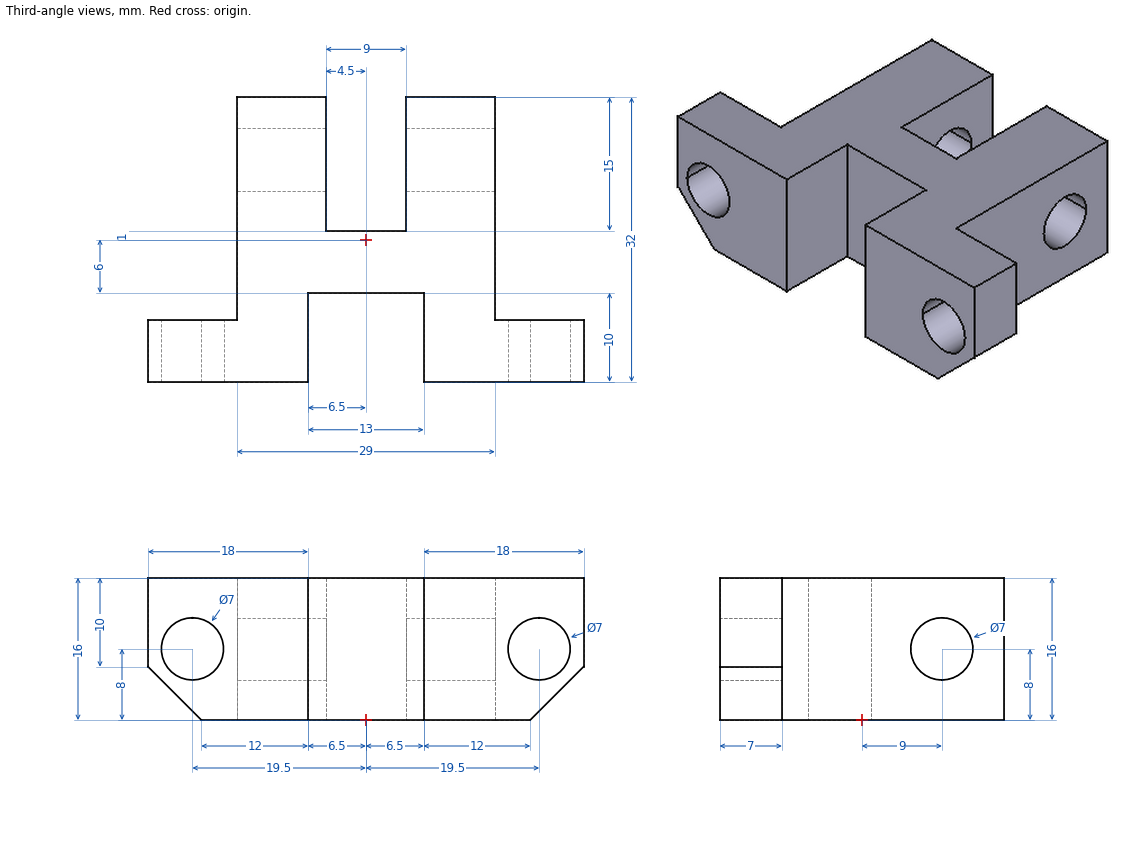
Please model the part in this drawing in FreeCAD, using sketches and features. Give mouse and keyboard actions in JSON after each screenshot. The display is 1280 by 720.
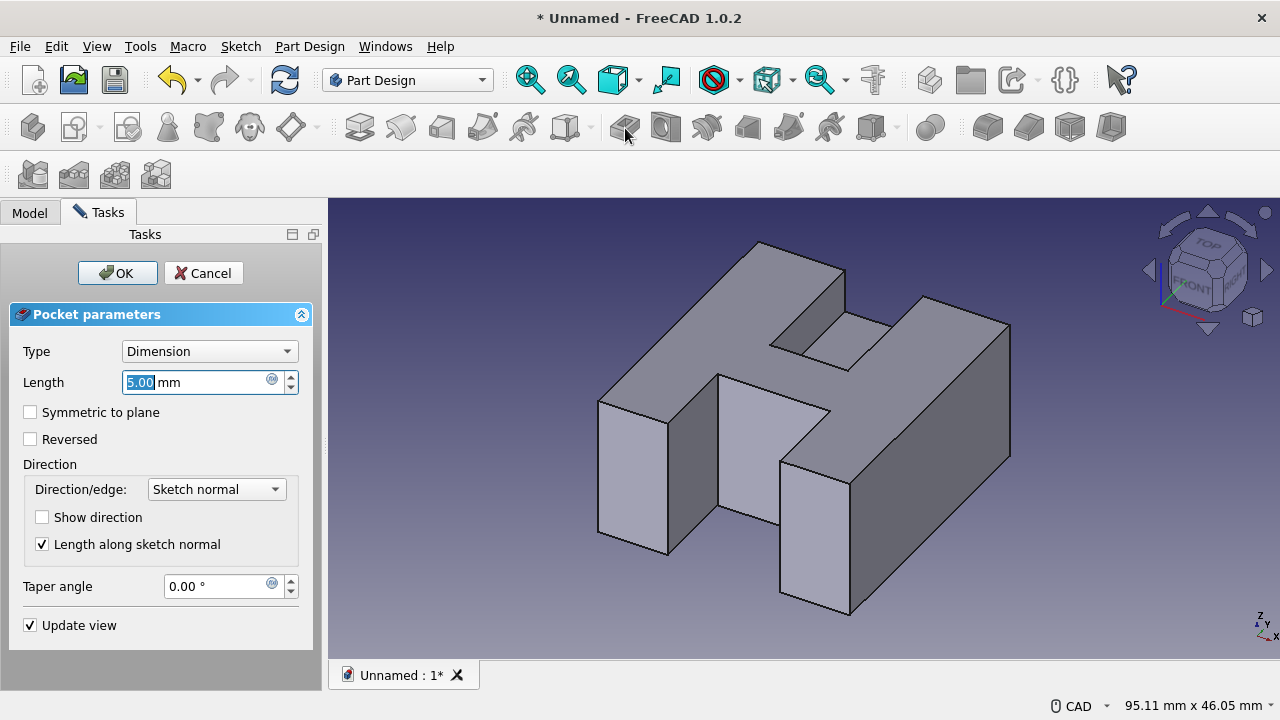
{"action": "left_click", "coordinate": [210, 352]}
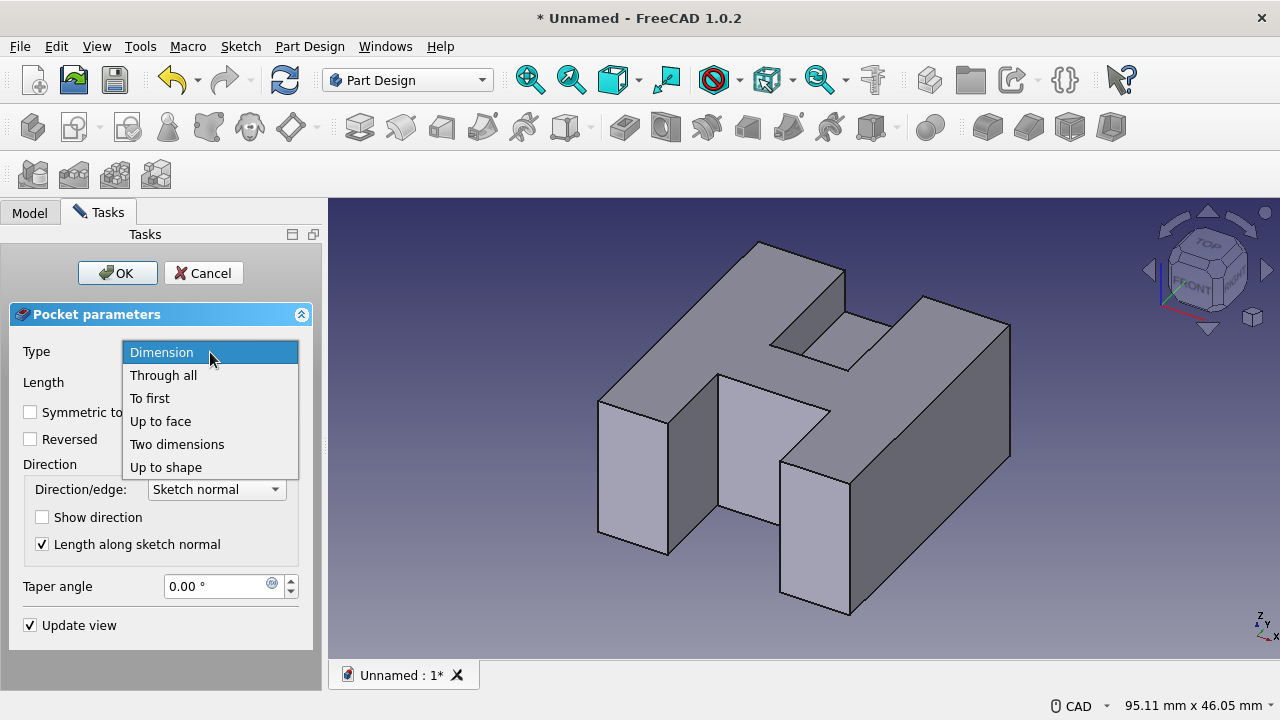
{"action": "left_click", "coordinate": [208, 376]}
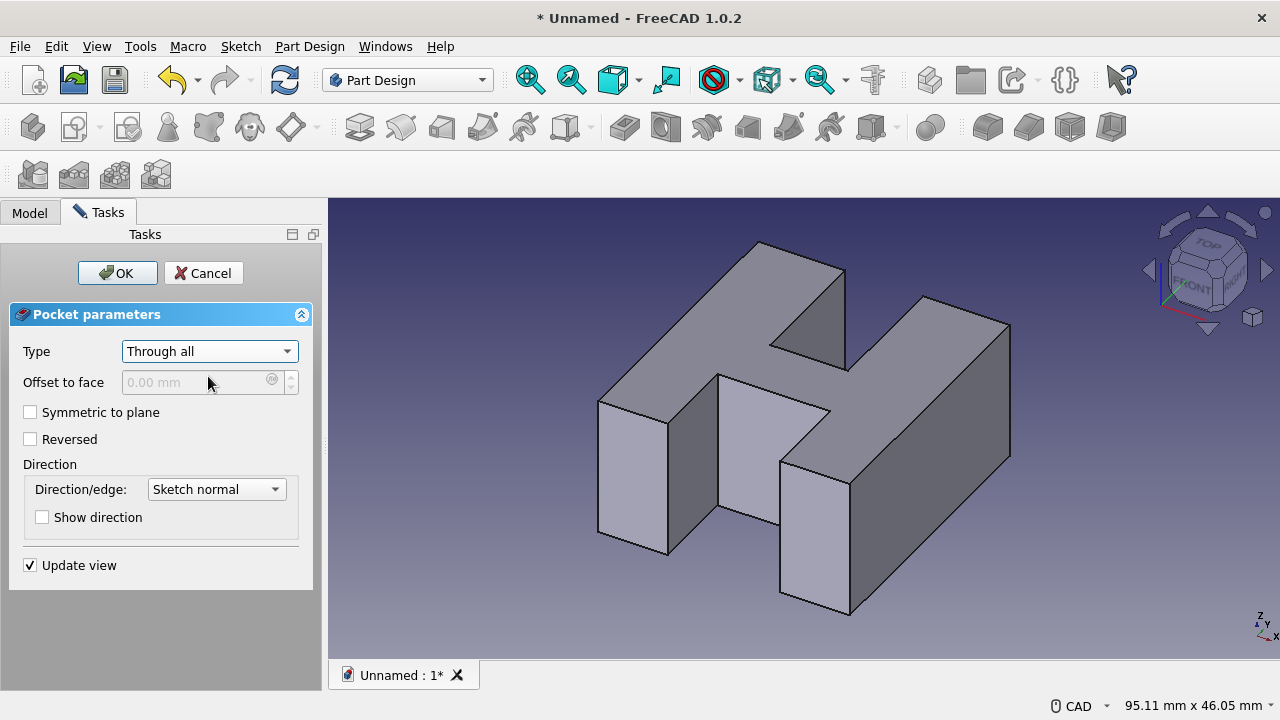
{"action": "left_click", "coordinate": [118, 273]}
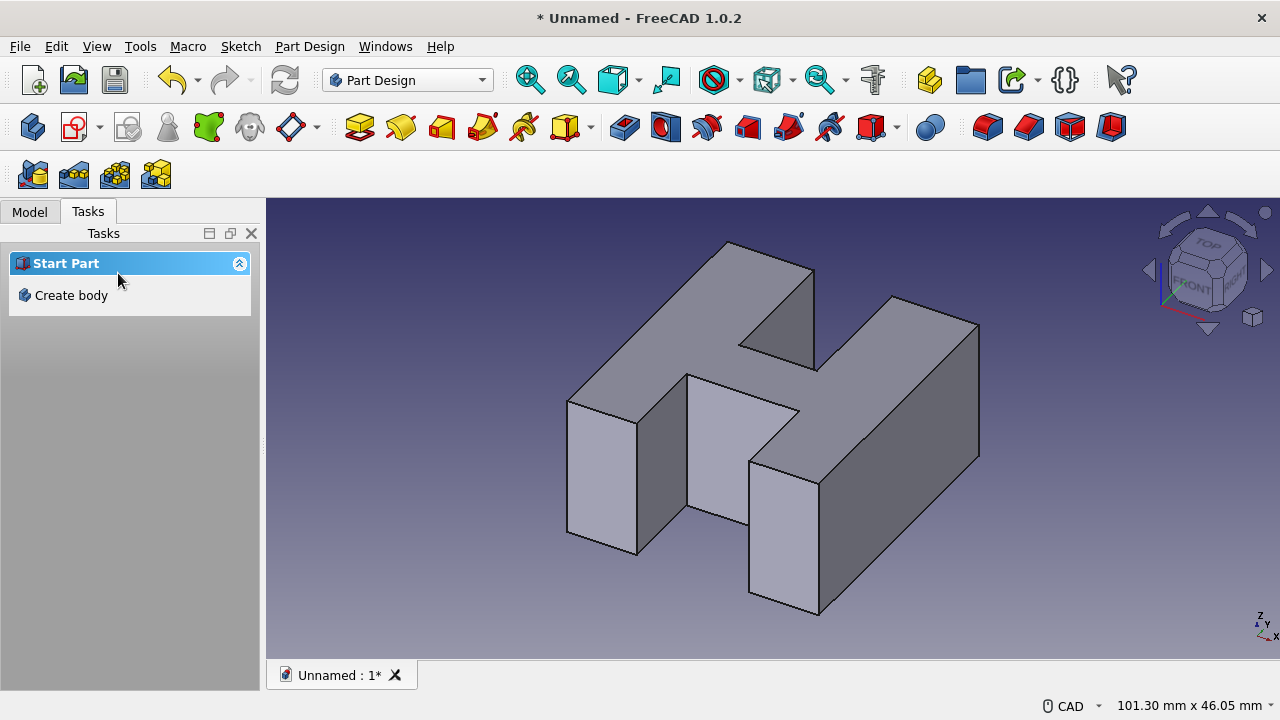
{"action": "left_click", "coordinate": [922, 446]}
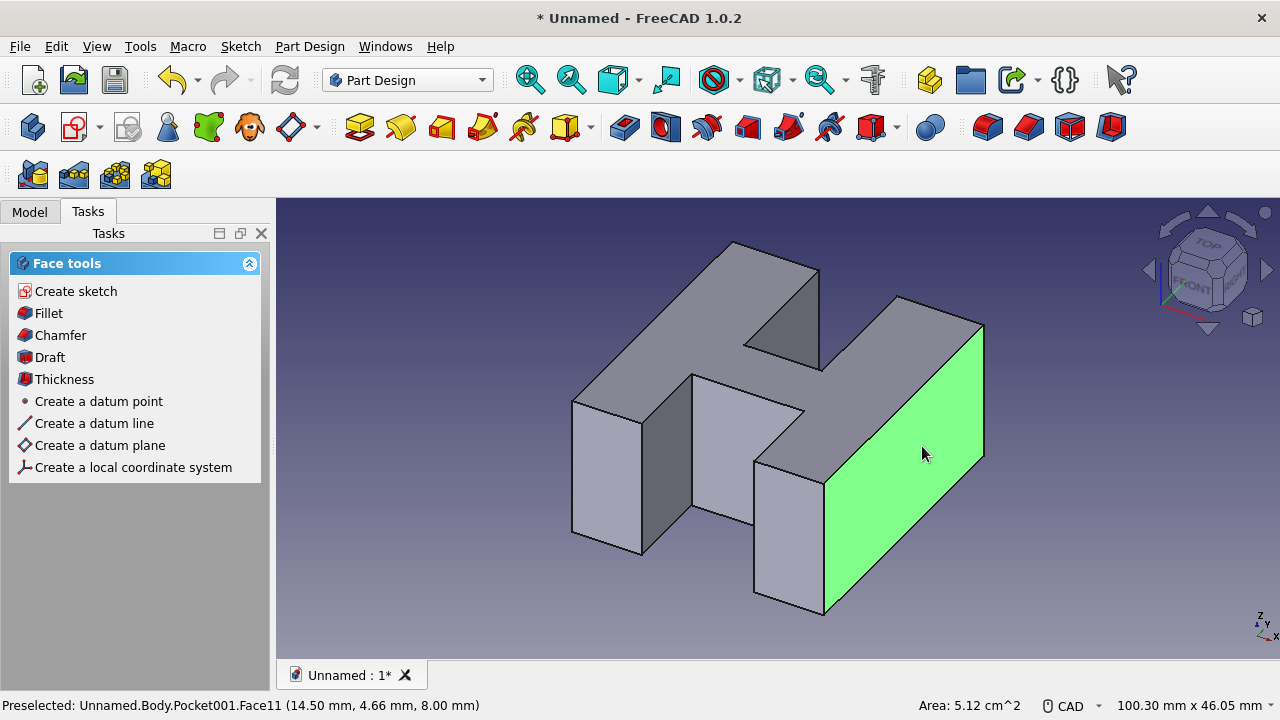
{"action": "left_click", "coordinate": [74, 128]}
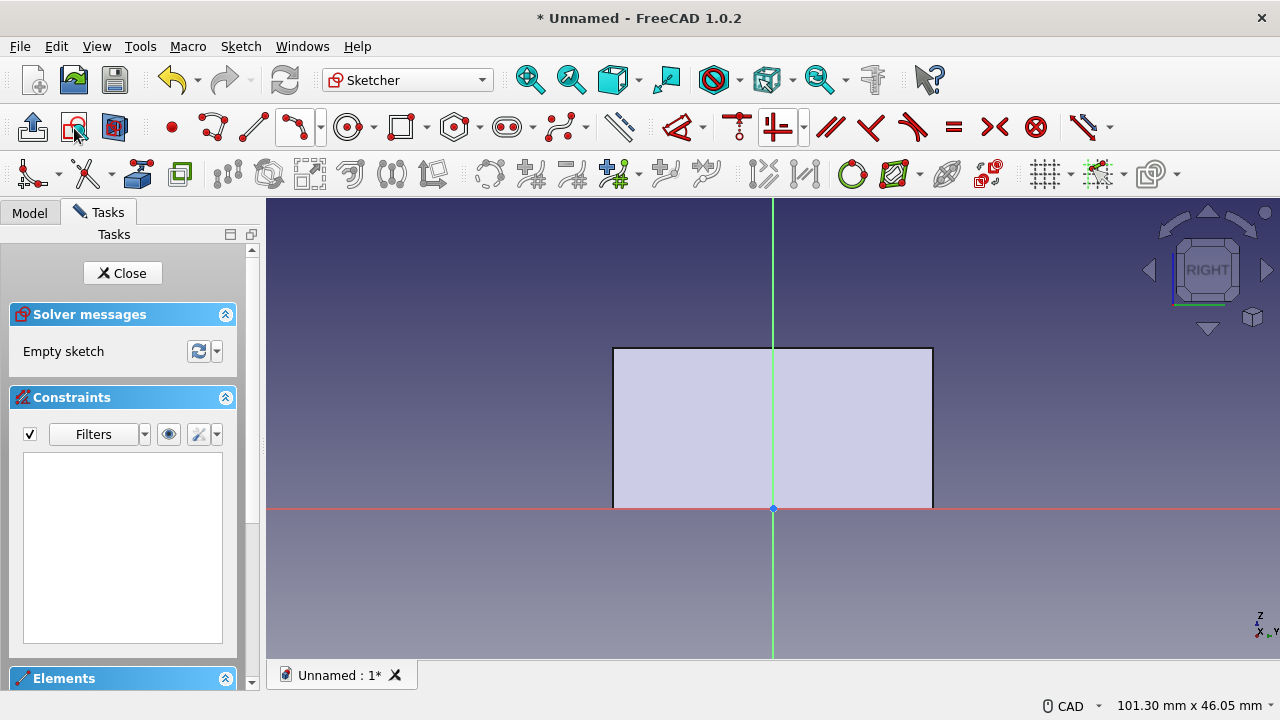
{"action": "scroll", "coordinate": [912, 464], "scroll_direction": "up", "scroll_amount": 5}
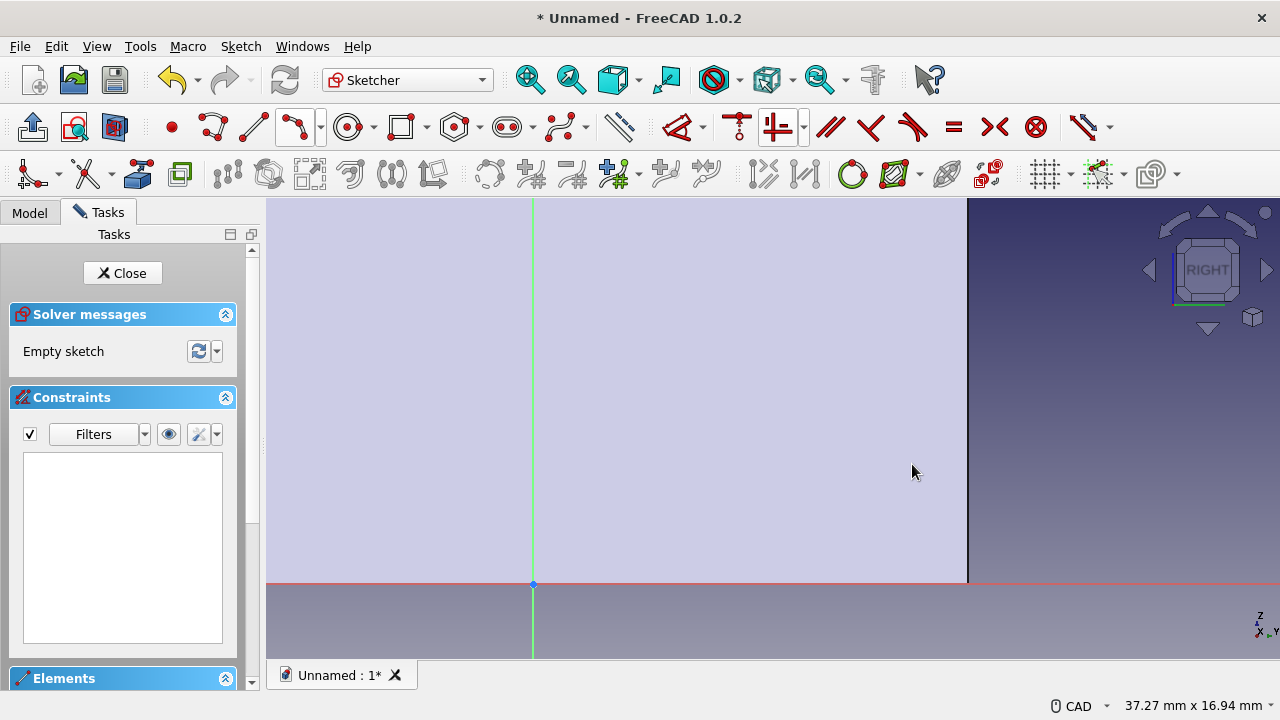
{"action": "left_click", "coordinate": [348, 128]}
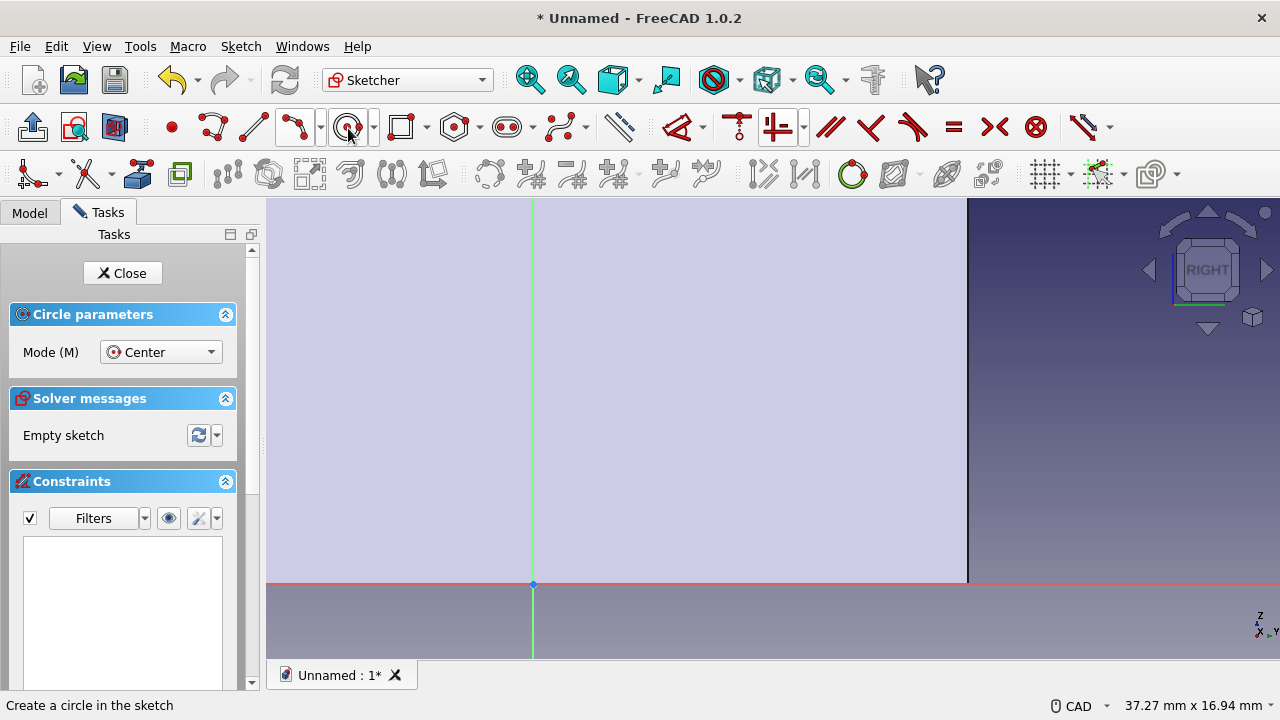
{"action": "left_click", "coordinate": [778, 367]}
{"action": "mouse_move", "coordinate": [845, 299]}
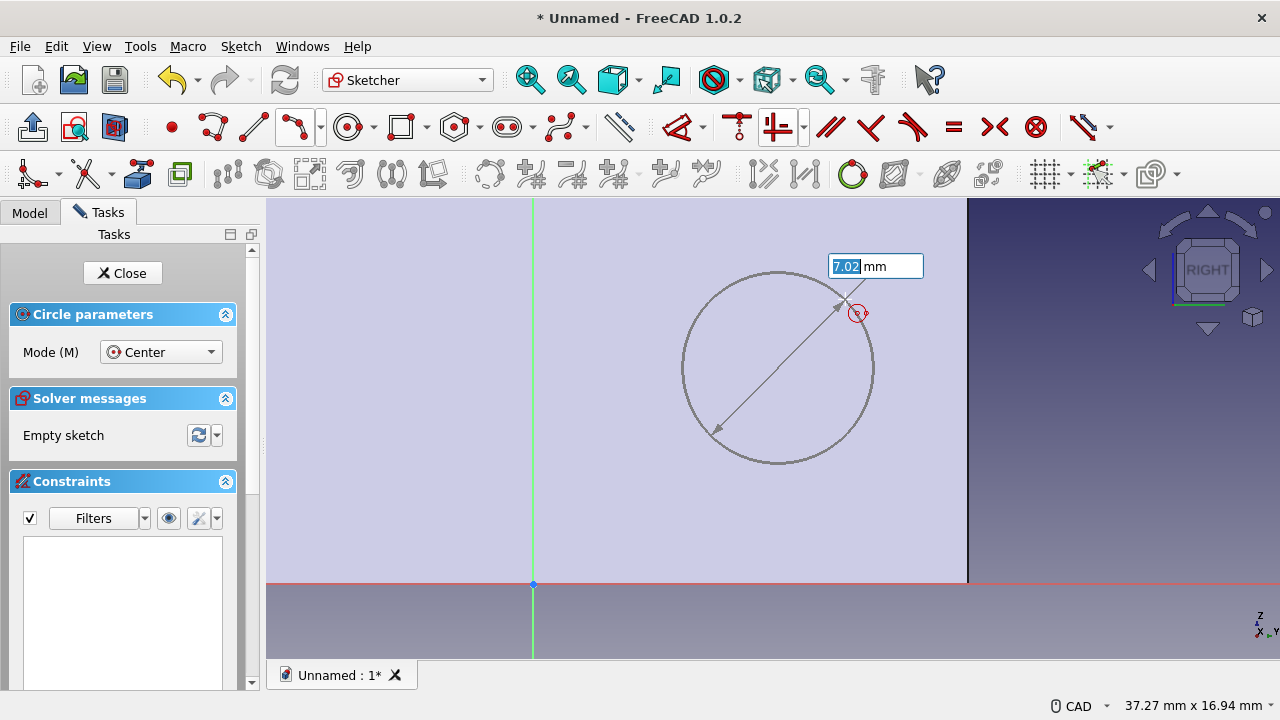
{"action": "type", "text": "7"}
{"action": "key", "text": "Return"}
{"action": "key", "text": "Escape"}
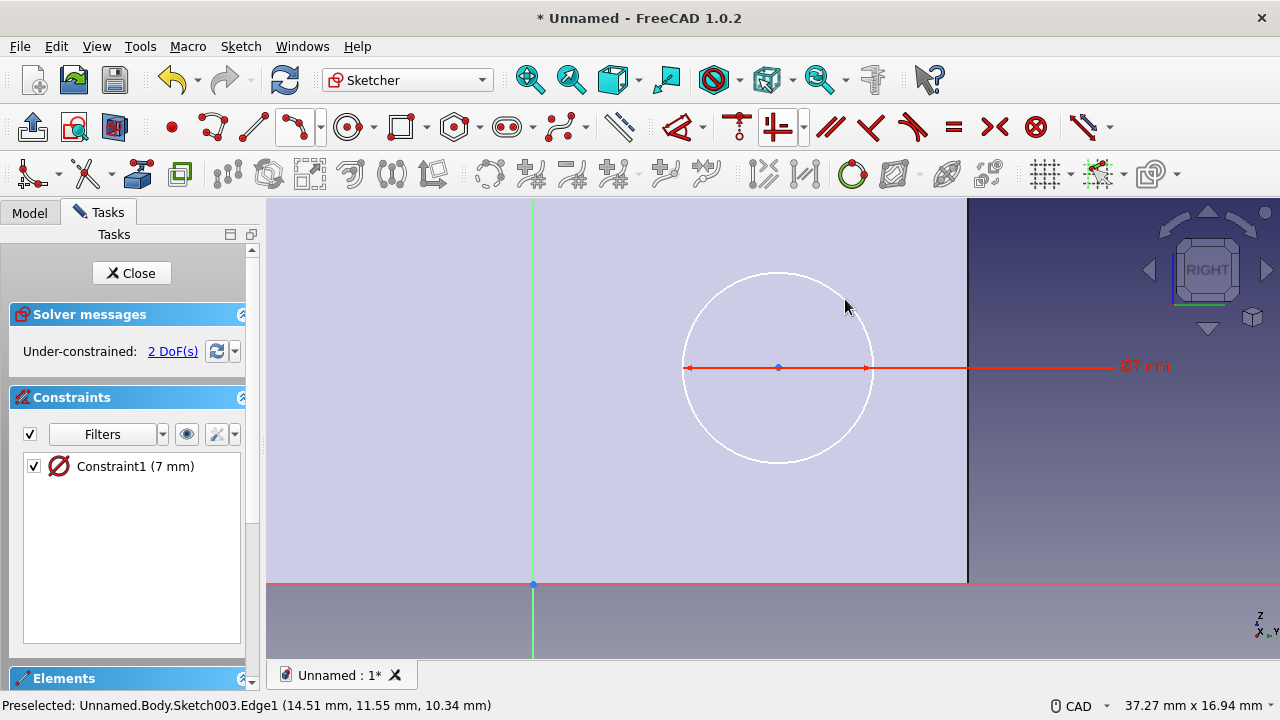
{"action": "left_click", "coordinate": [676, 128]}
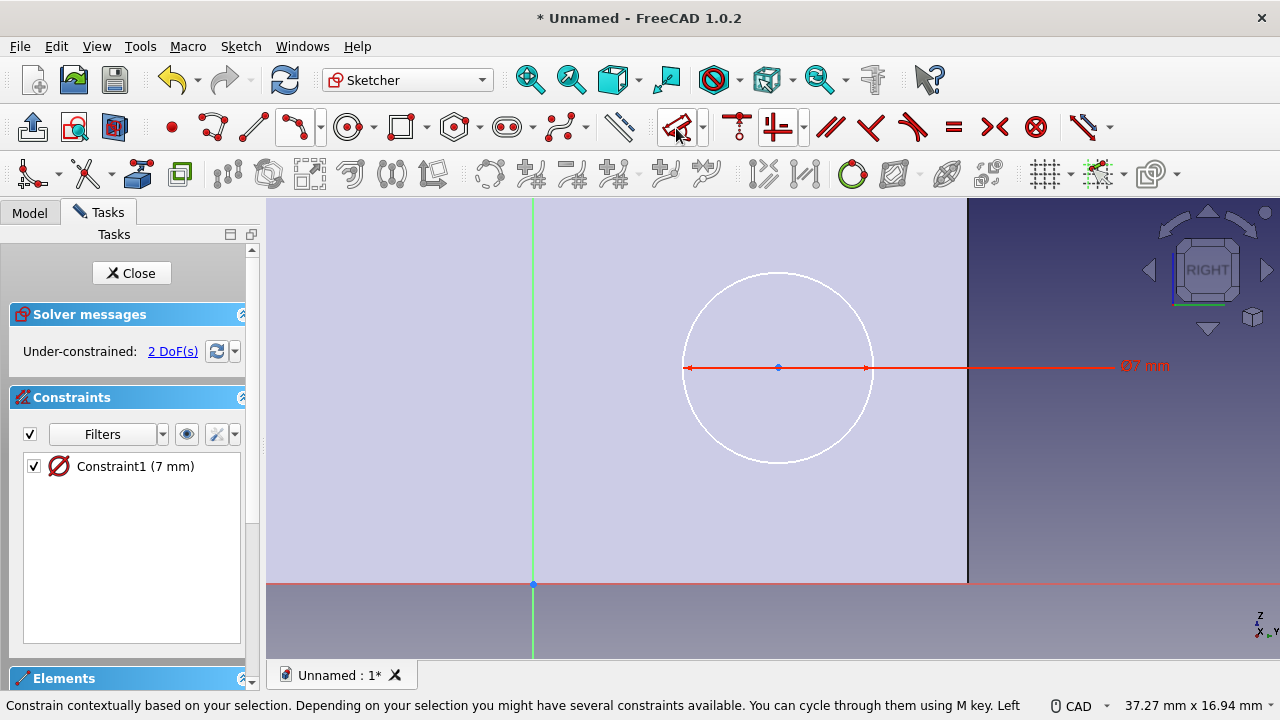
{"action": "left_click", "coordinate": [778, 368]}
{"action": "left_click", "coordinate": [656, 618]}